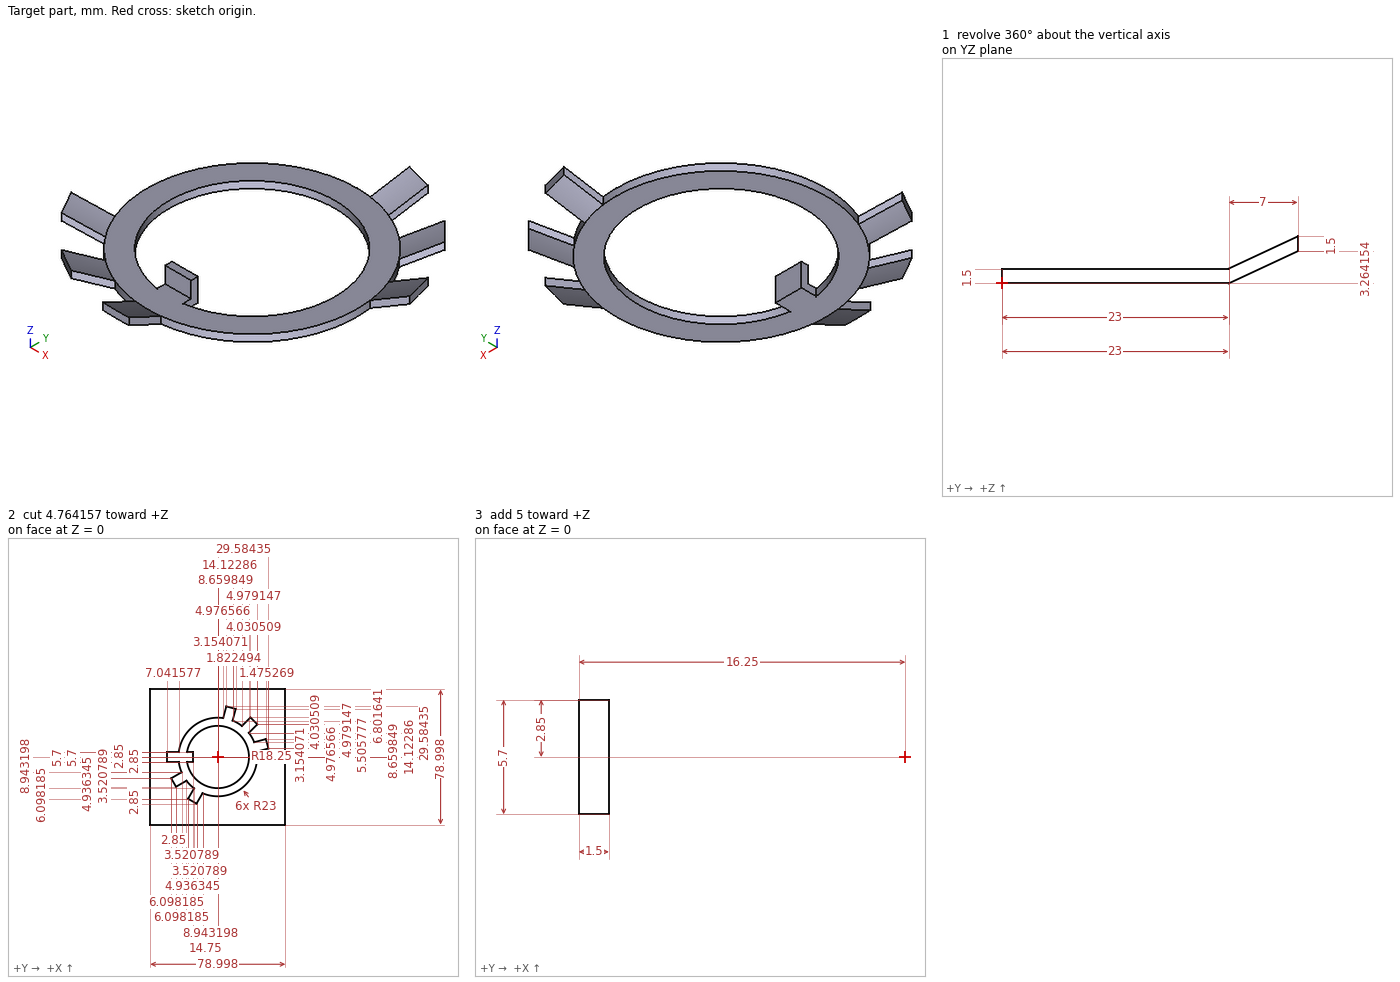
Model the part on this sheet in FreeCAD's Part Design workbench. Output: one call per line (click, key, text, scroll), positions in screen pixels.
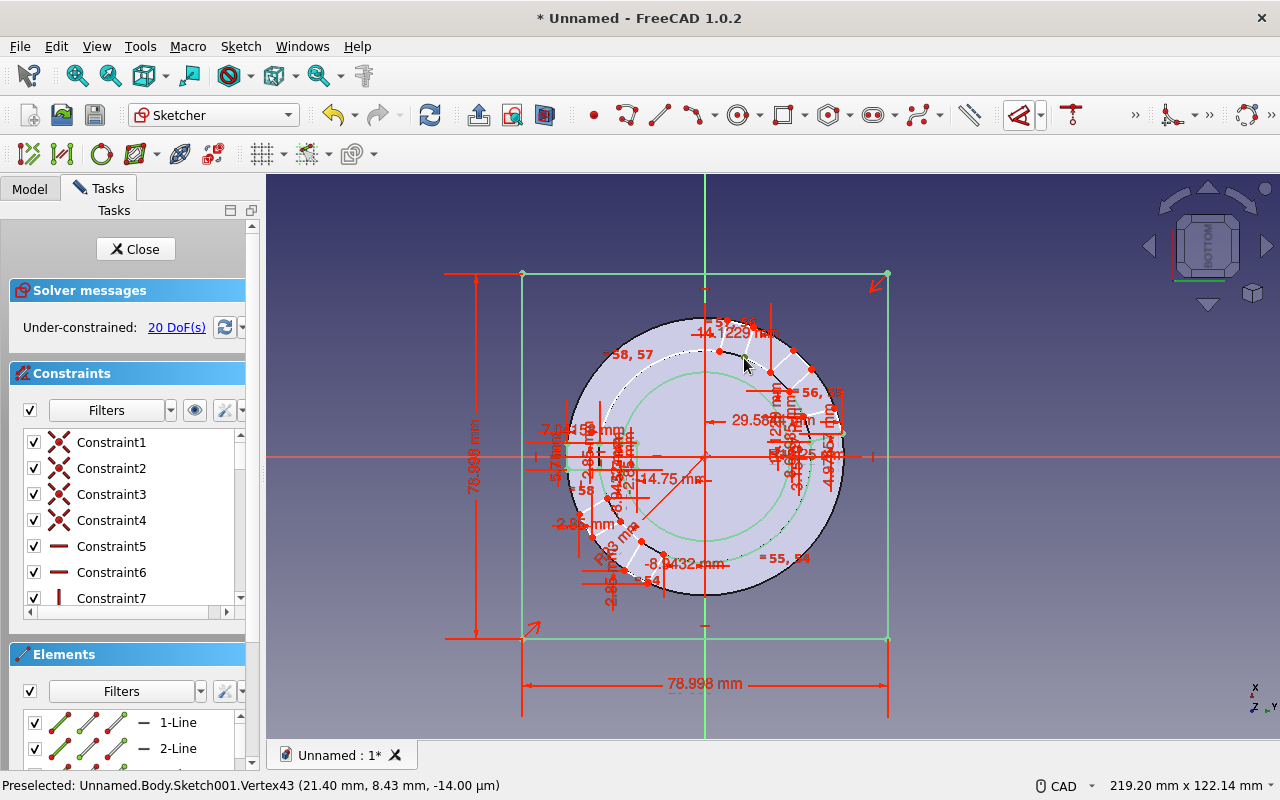
key(l)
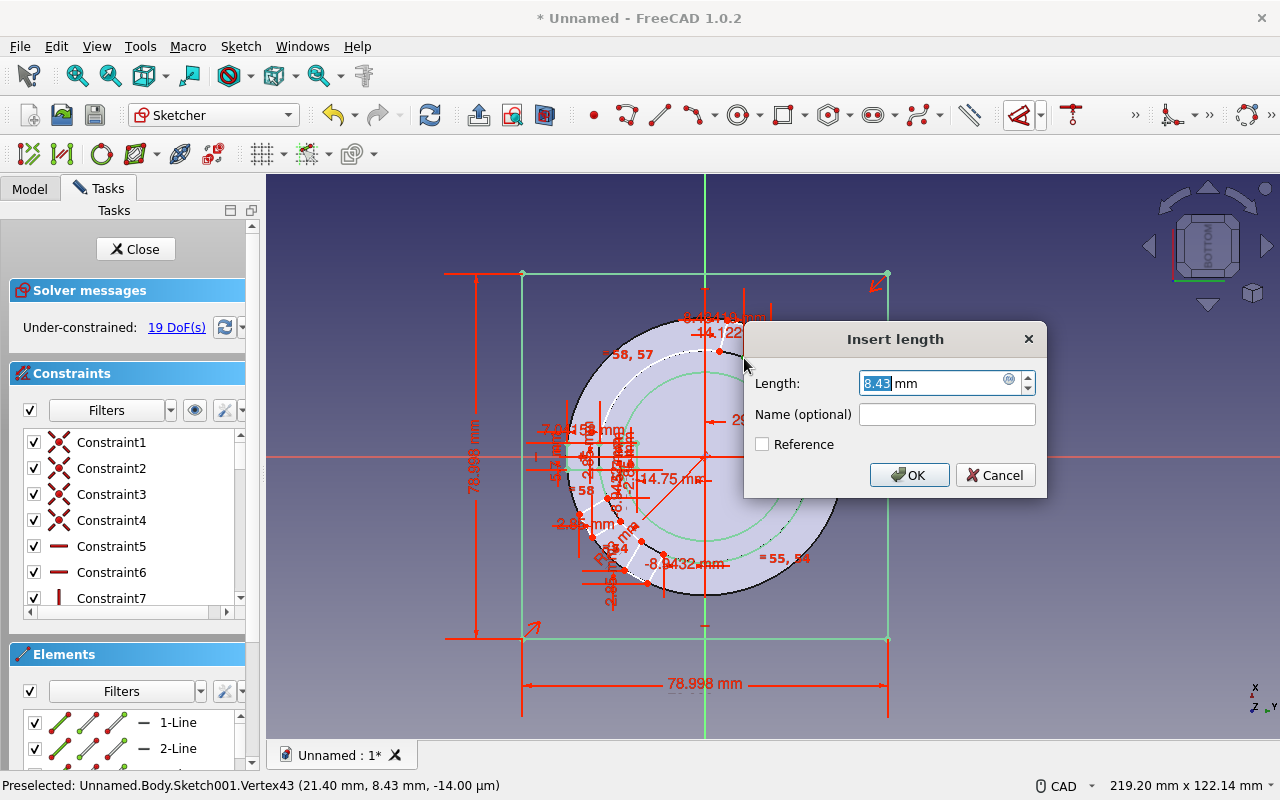
text(8.659849)
key(Return)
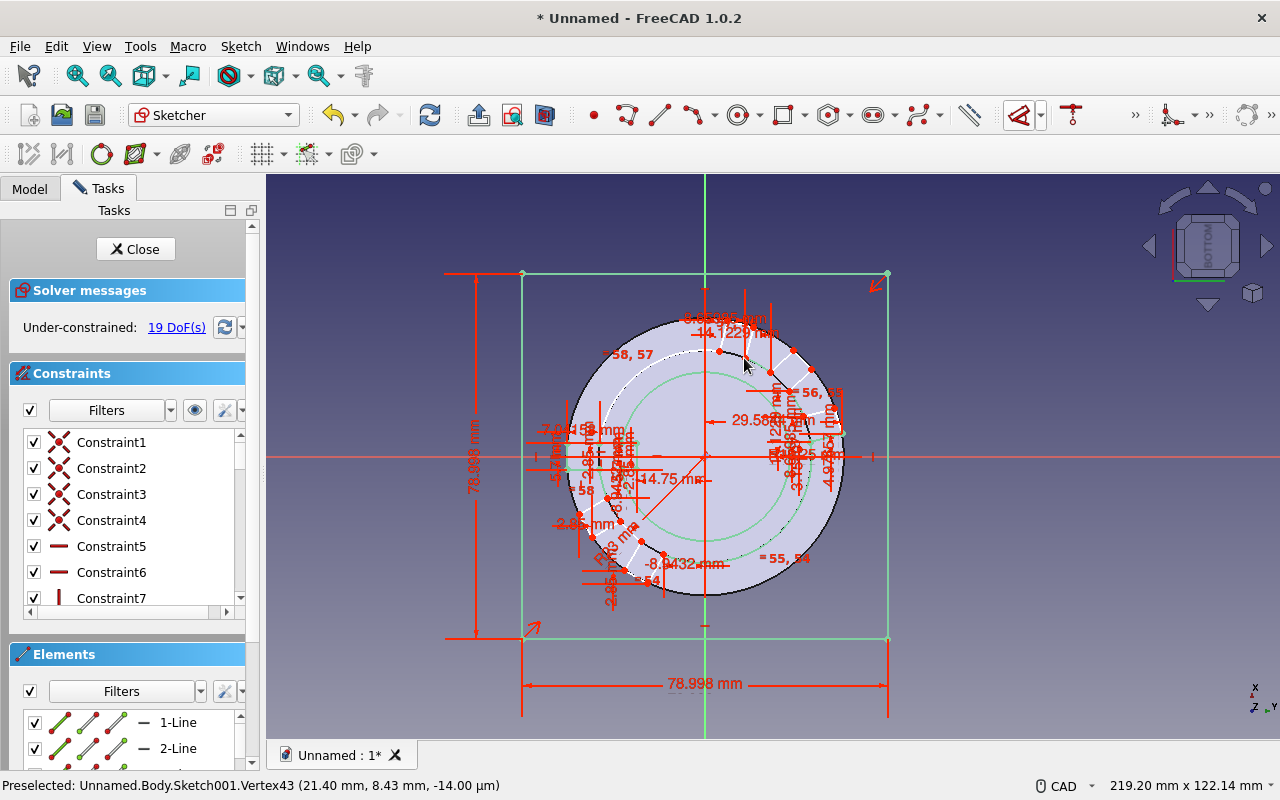
scroll(728, 321, up, 3)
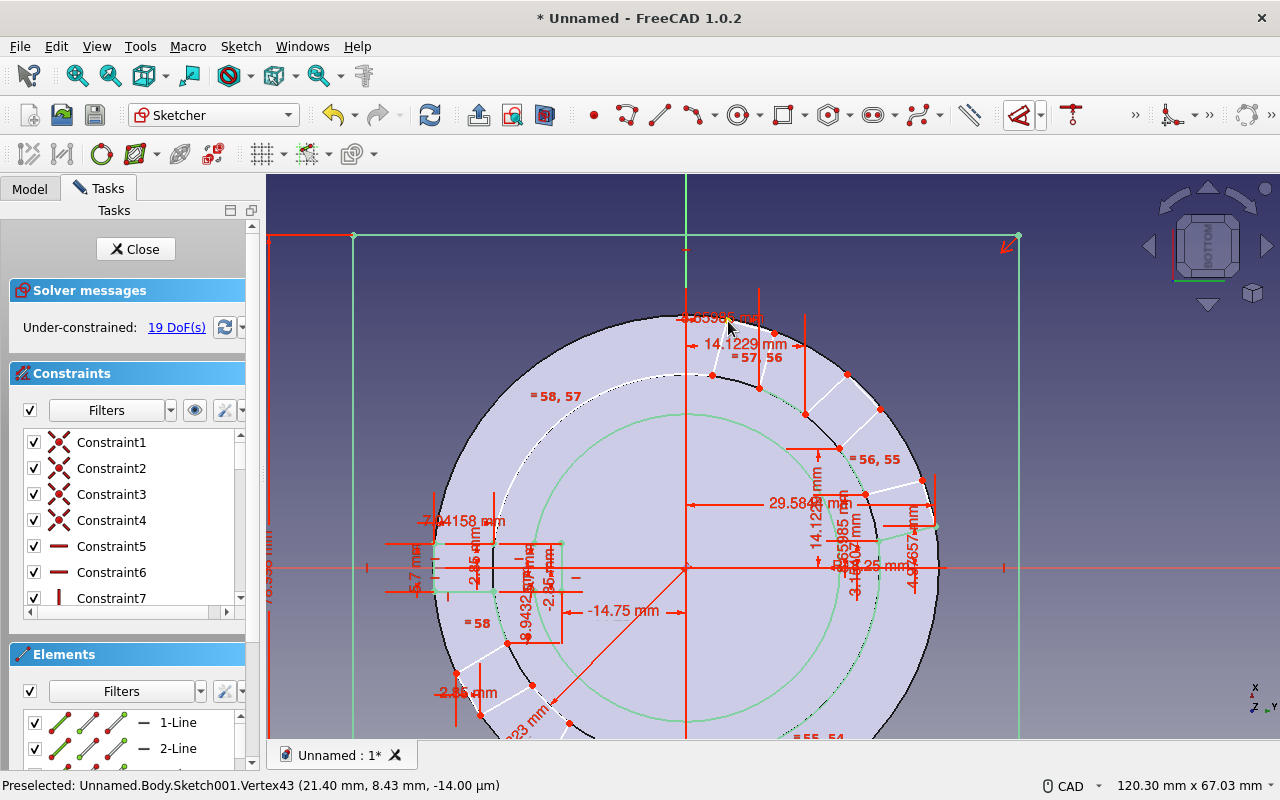
click(727, 320)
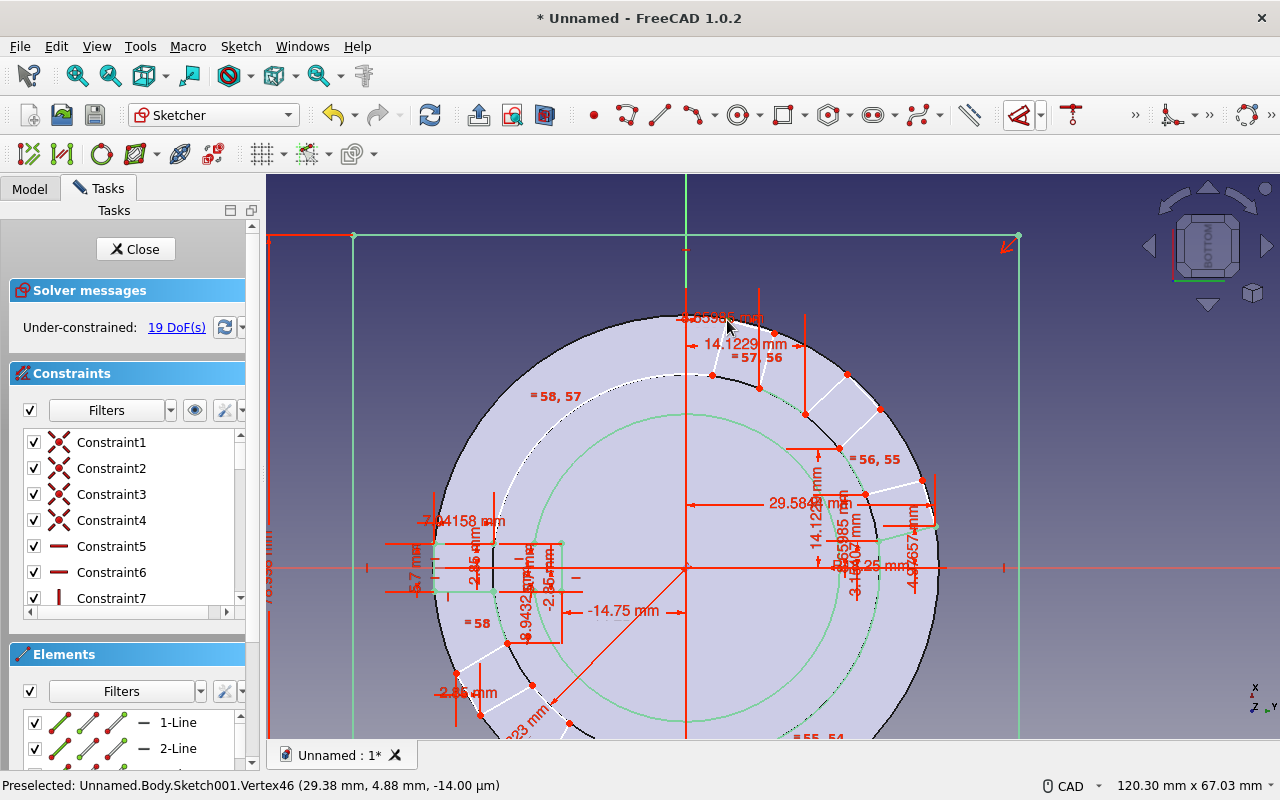
key(l)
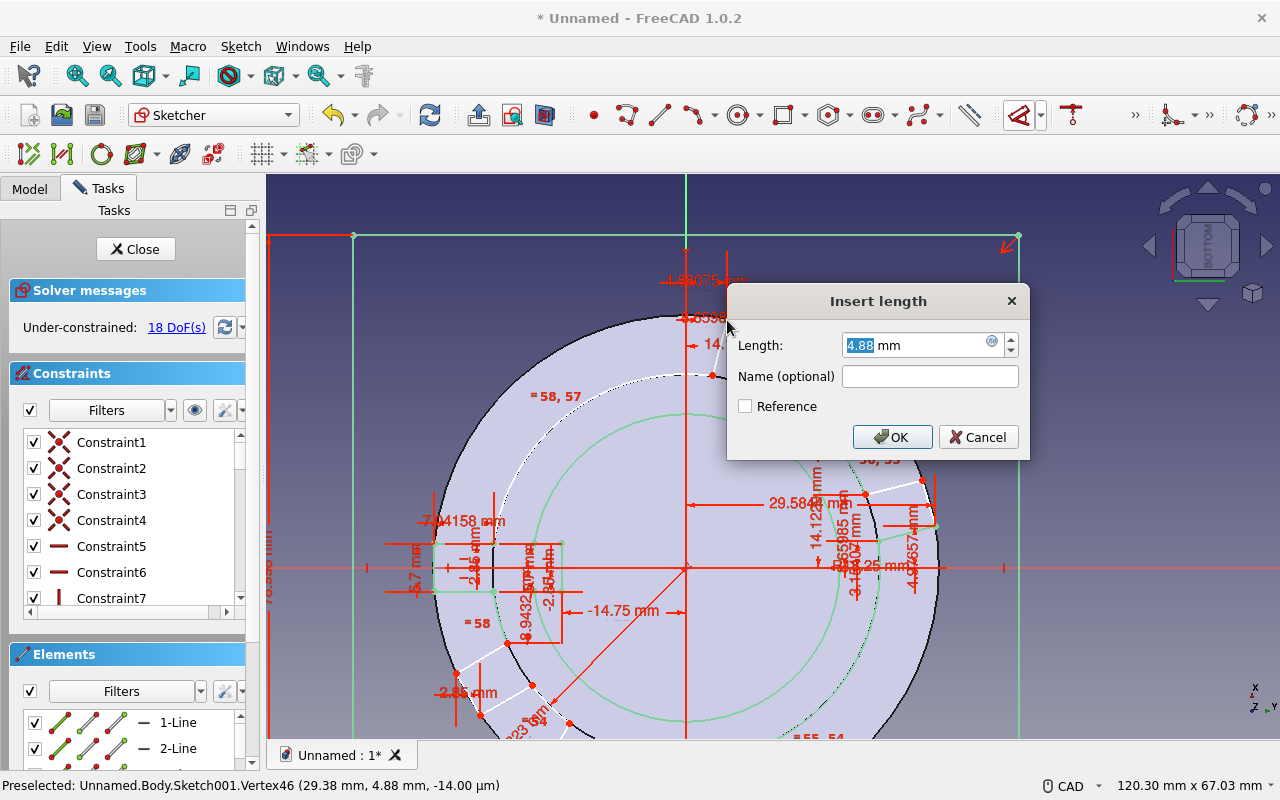
text(4.976566)
key(Return)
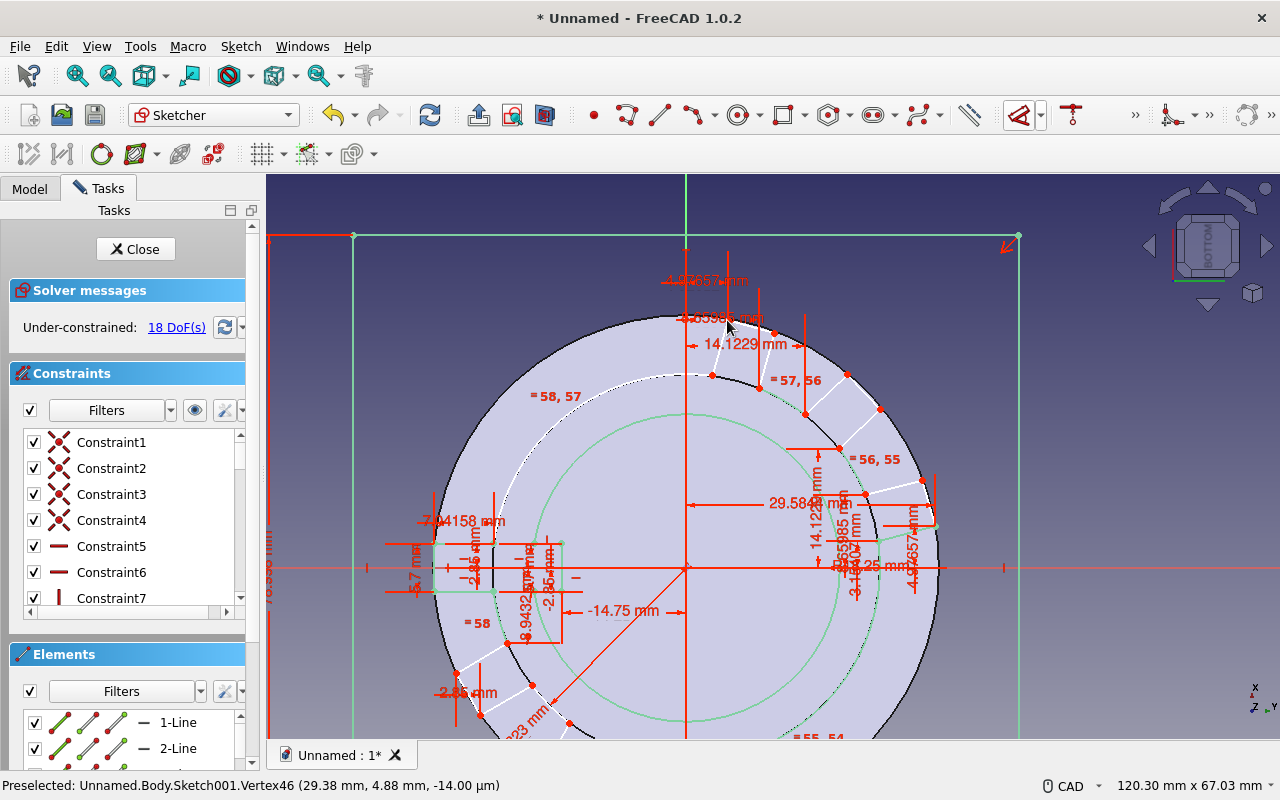
click(728, 320)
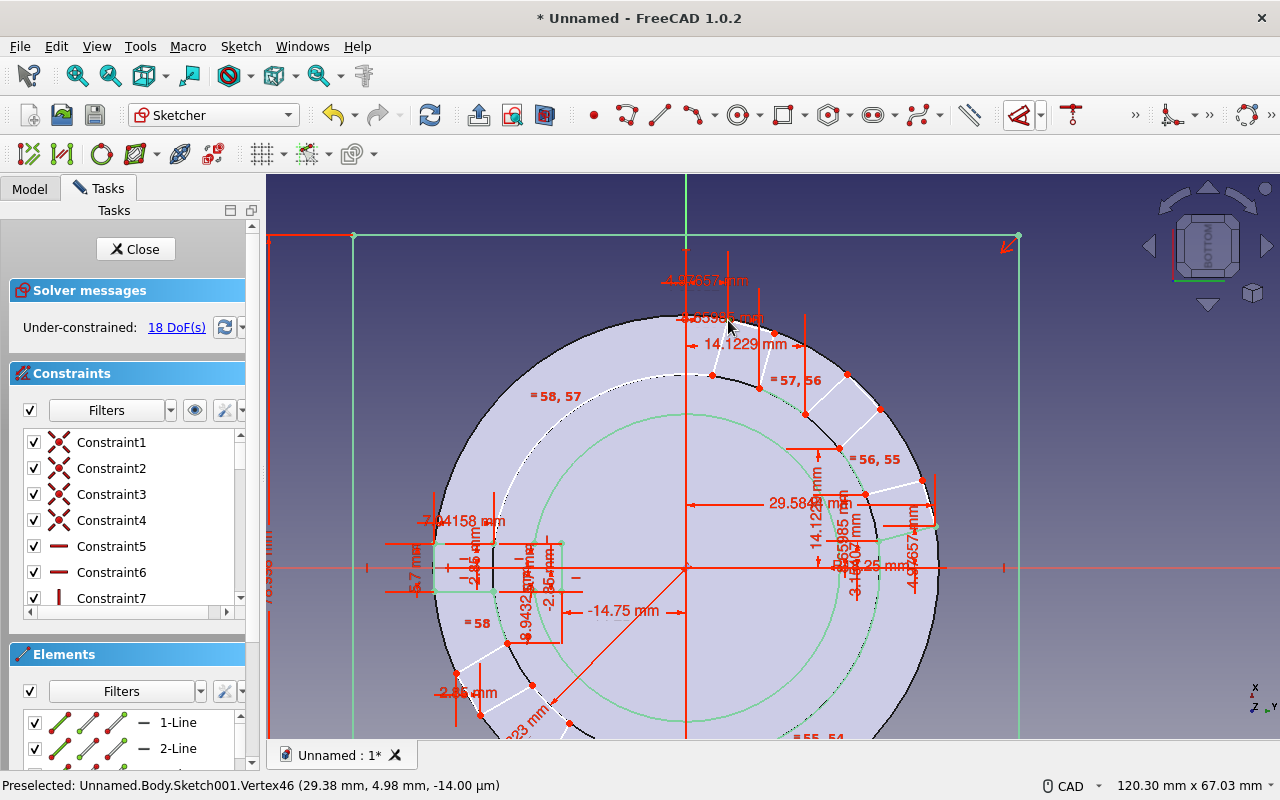
key(i)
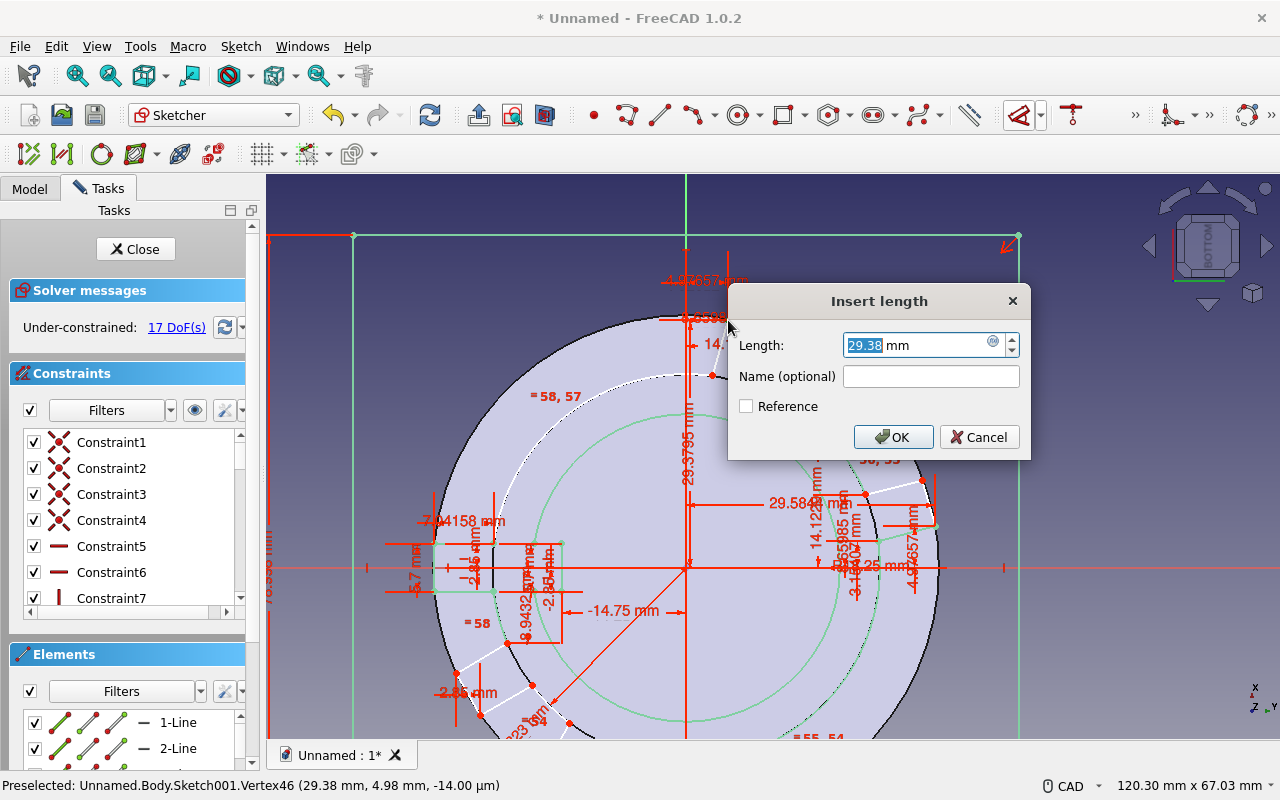
text(29.58435)
key(Return)